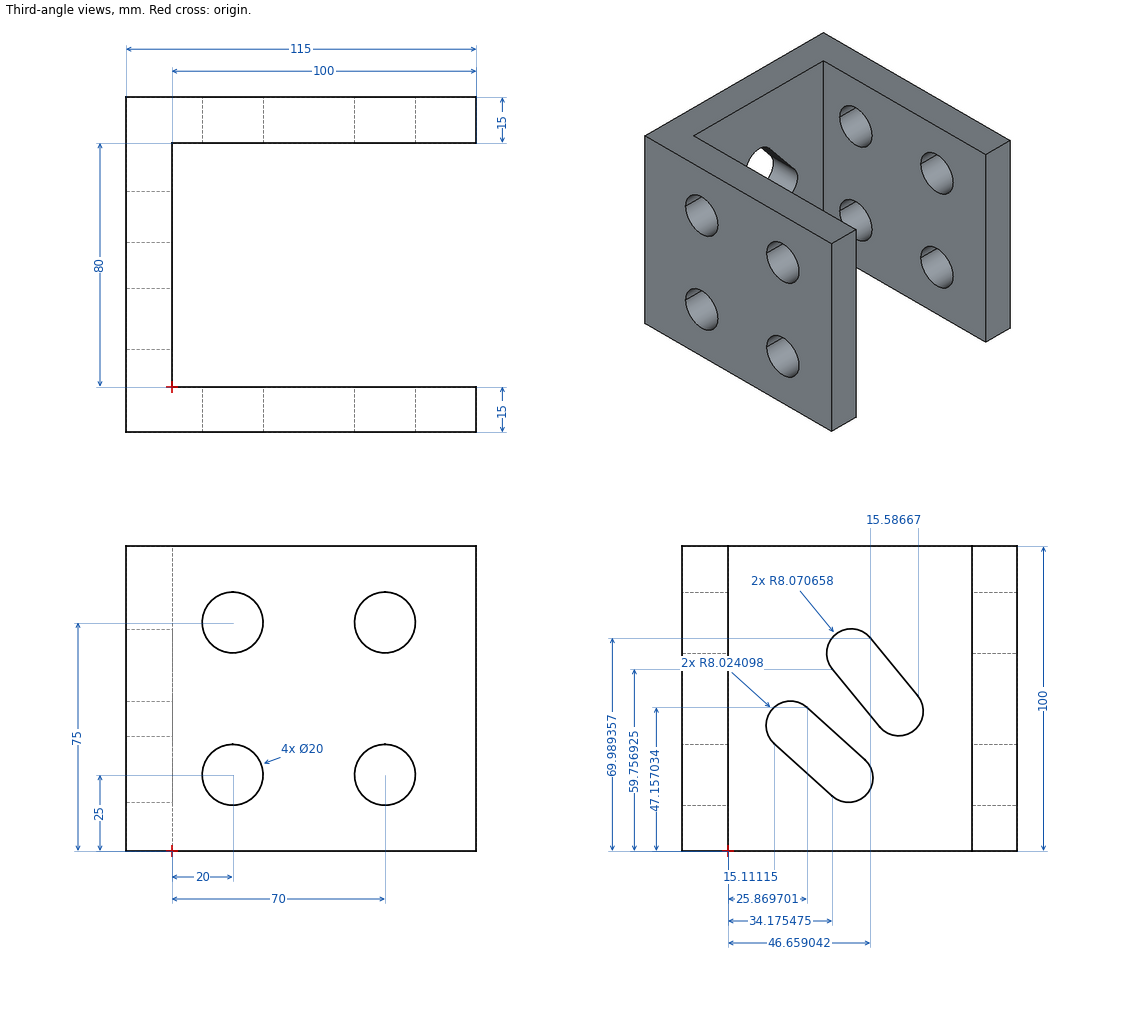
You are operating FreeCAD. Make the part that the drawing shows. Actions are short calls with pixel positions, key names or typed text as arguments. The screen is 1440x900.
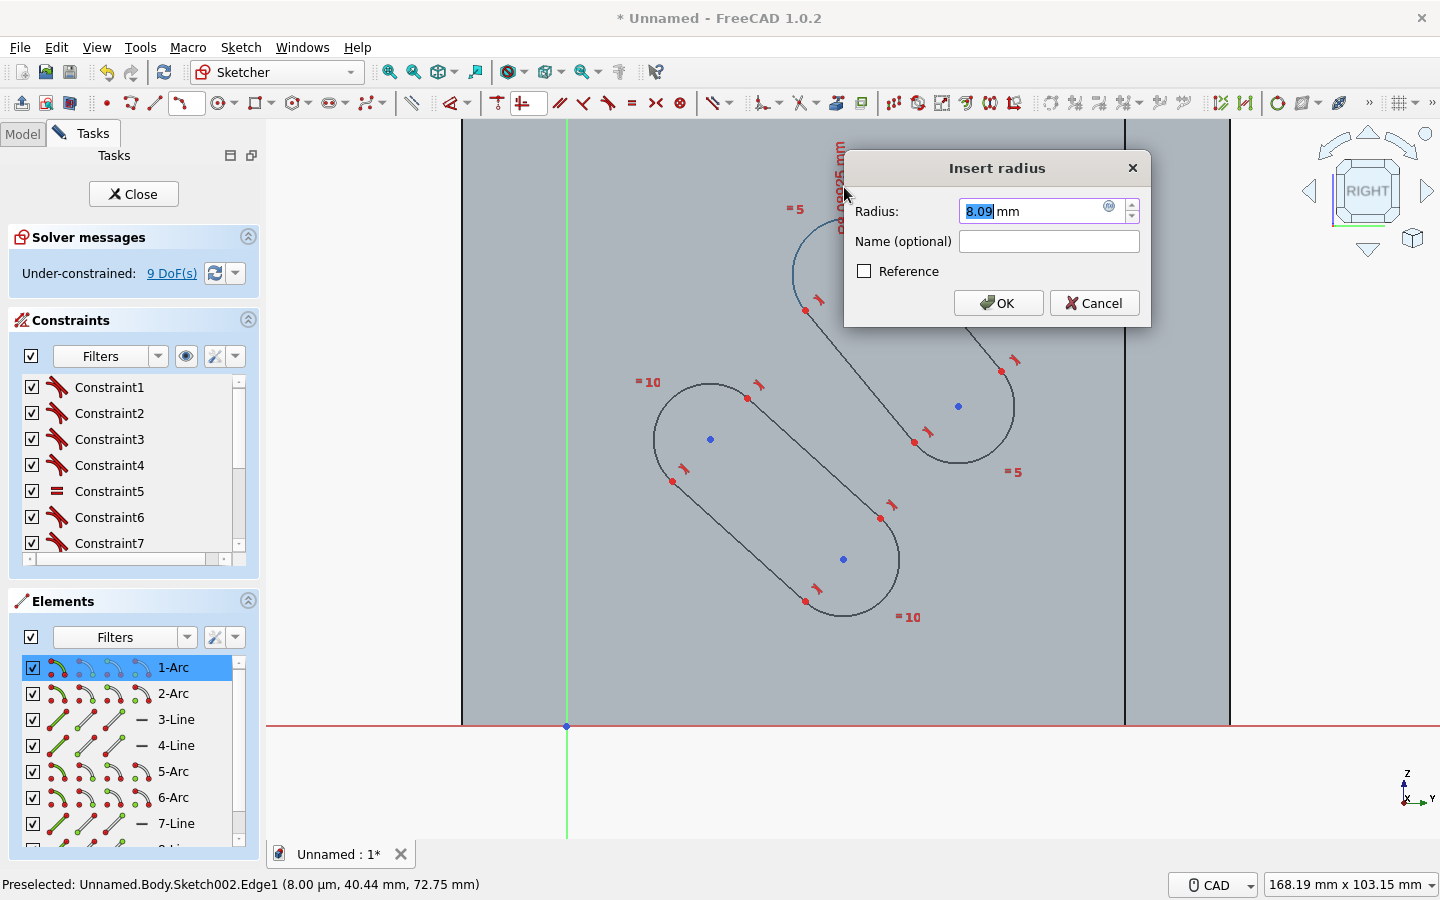
text(8.070658)
key(Return)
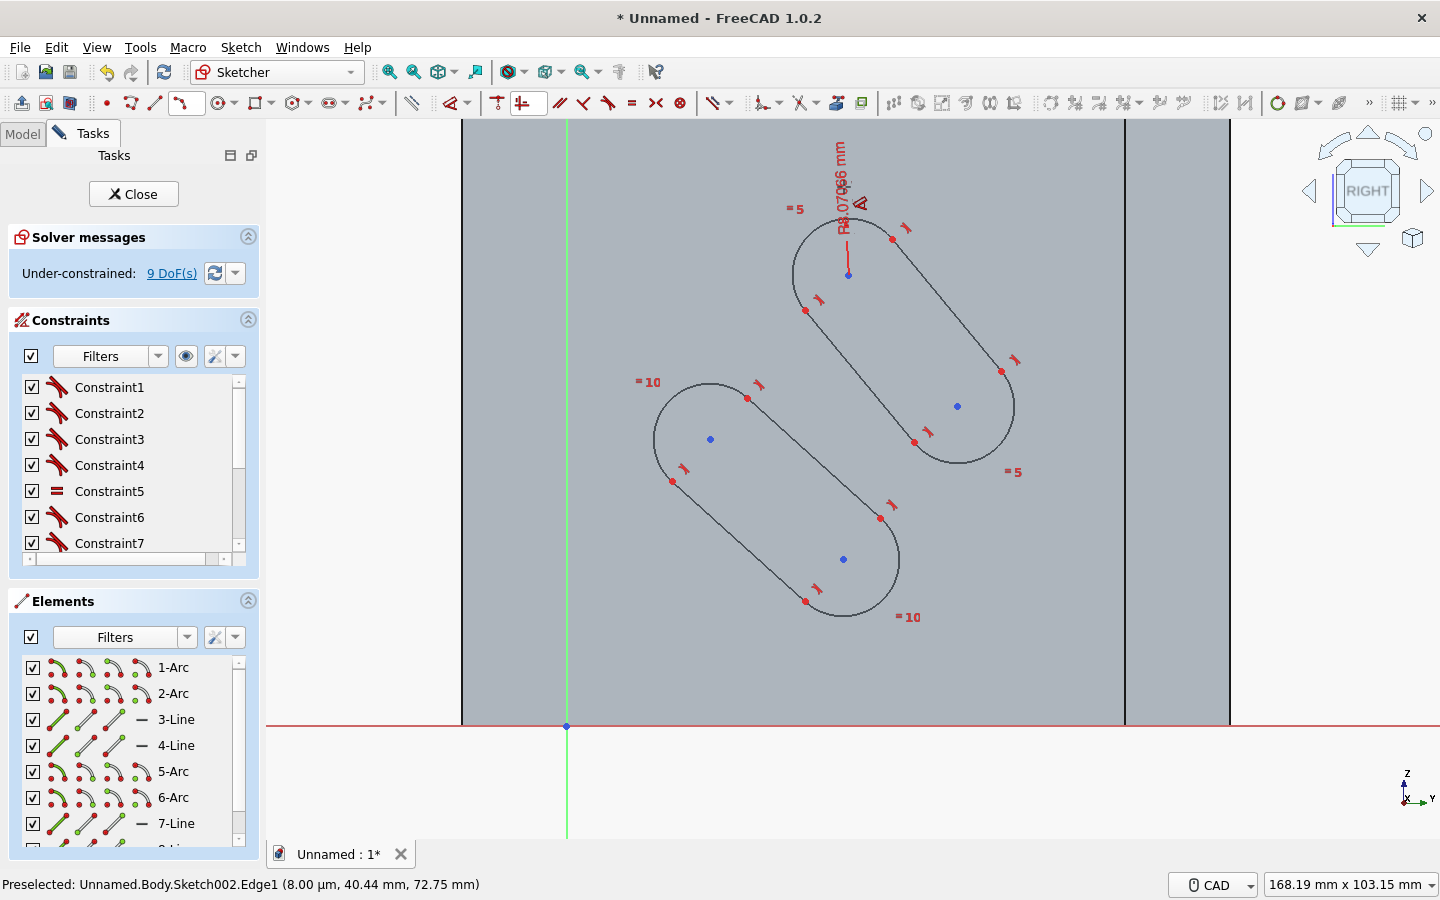
click(698, 385)
click(691, 354)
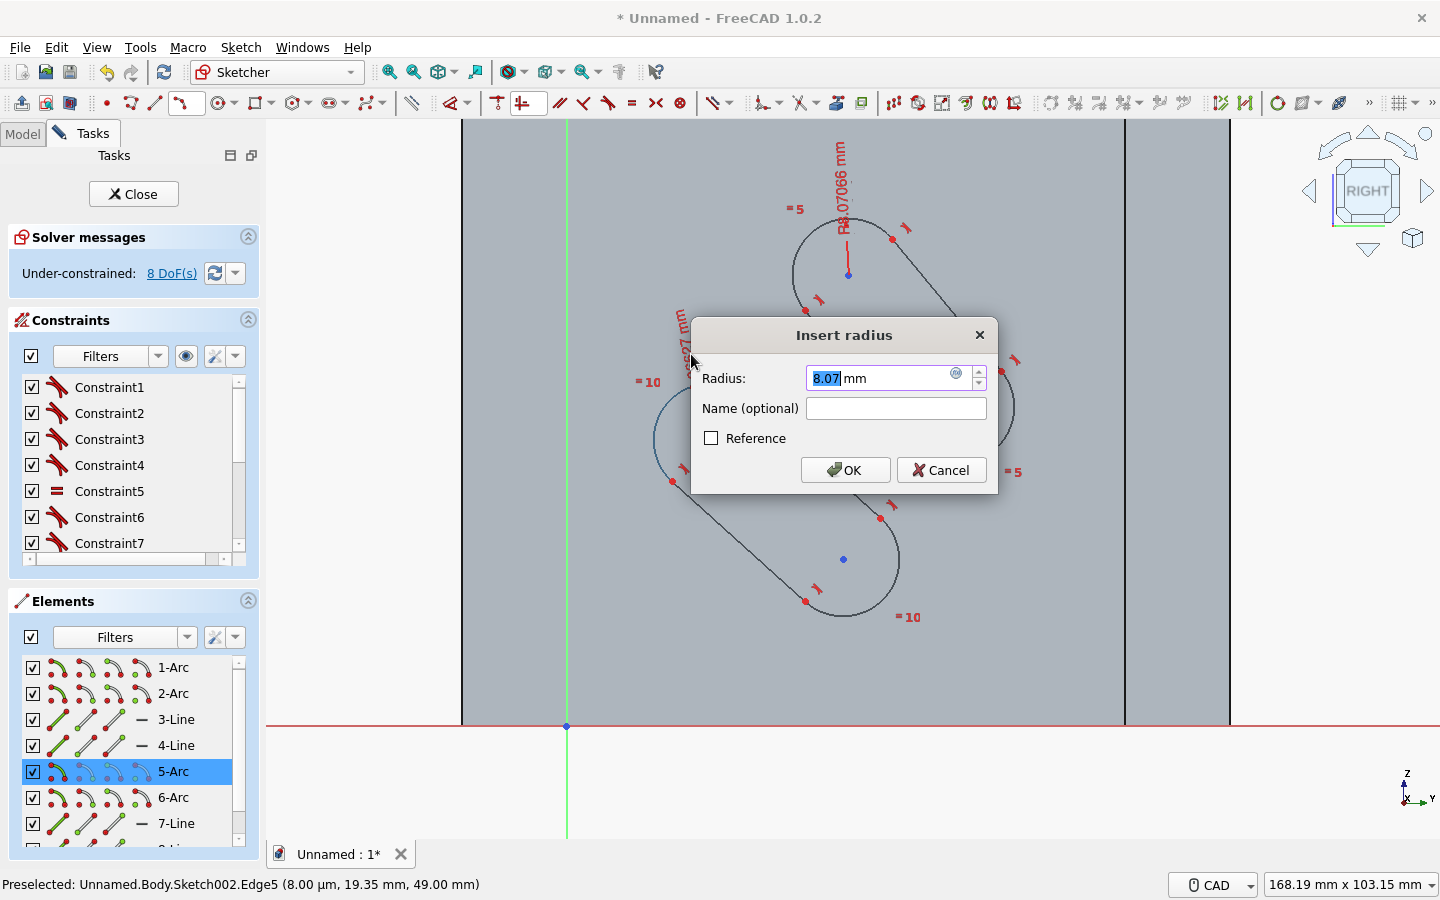
text(8.024098)
key(Return)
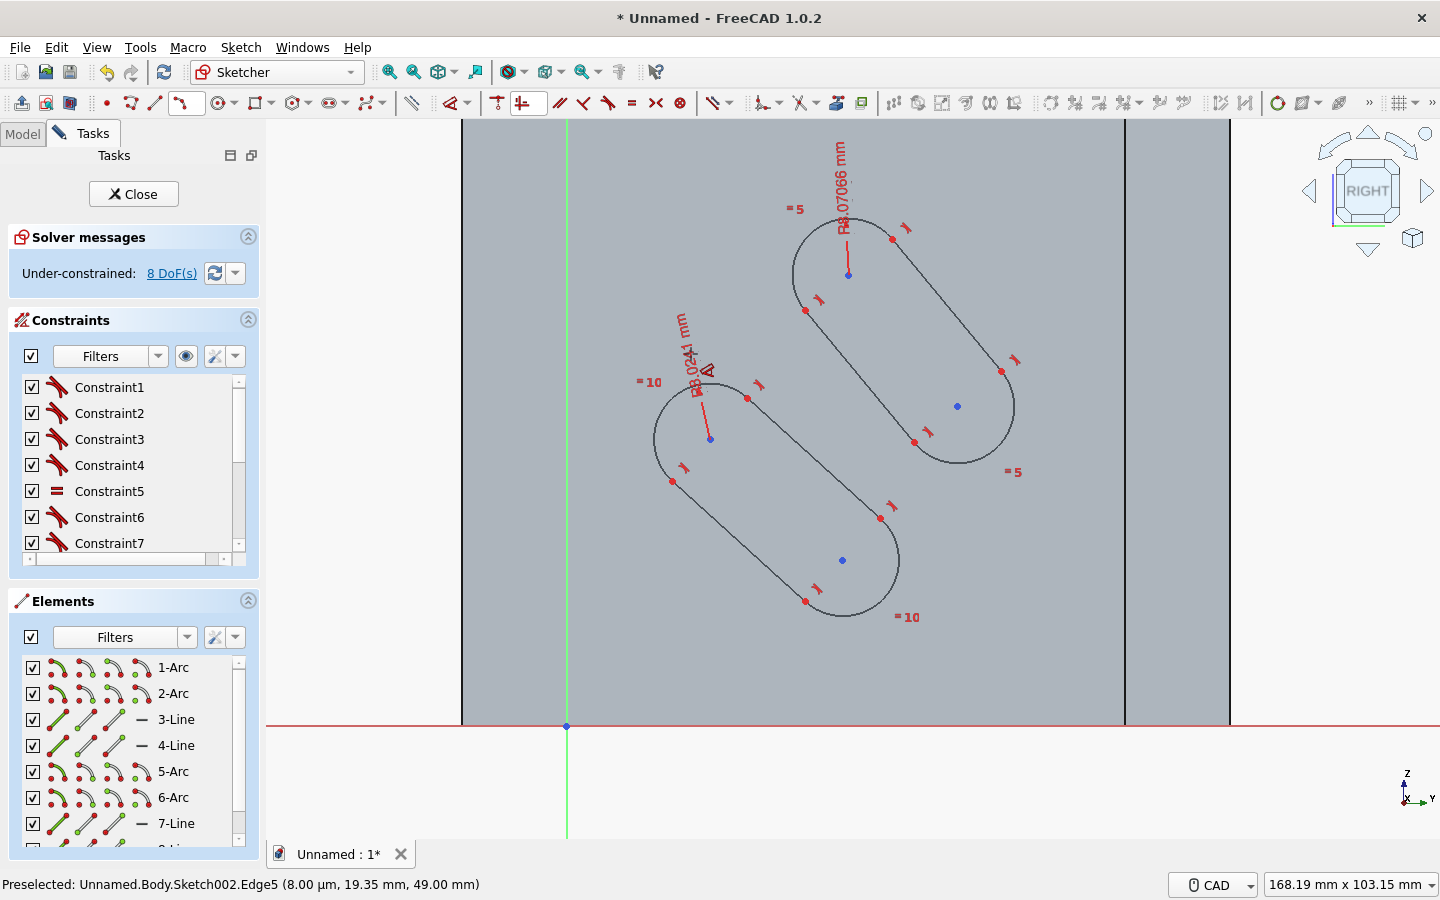
click(672, 481)
click(620, 760)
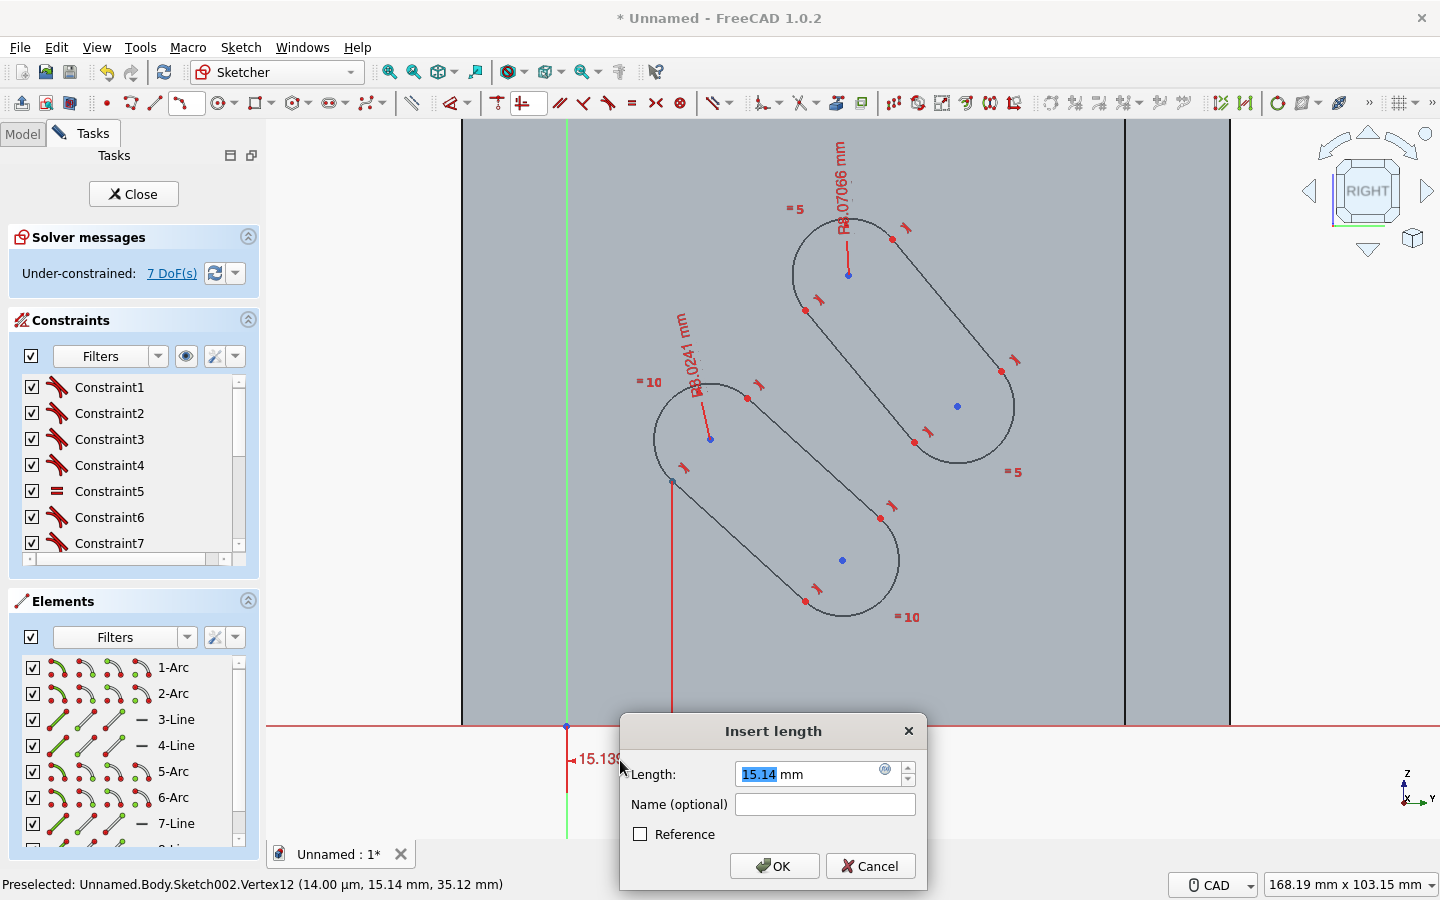
text(15.11115)
key(Return)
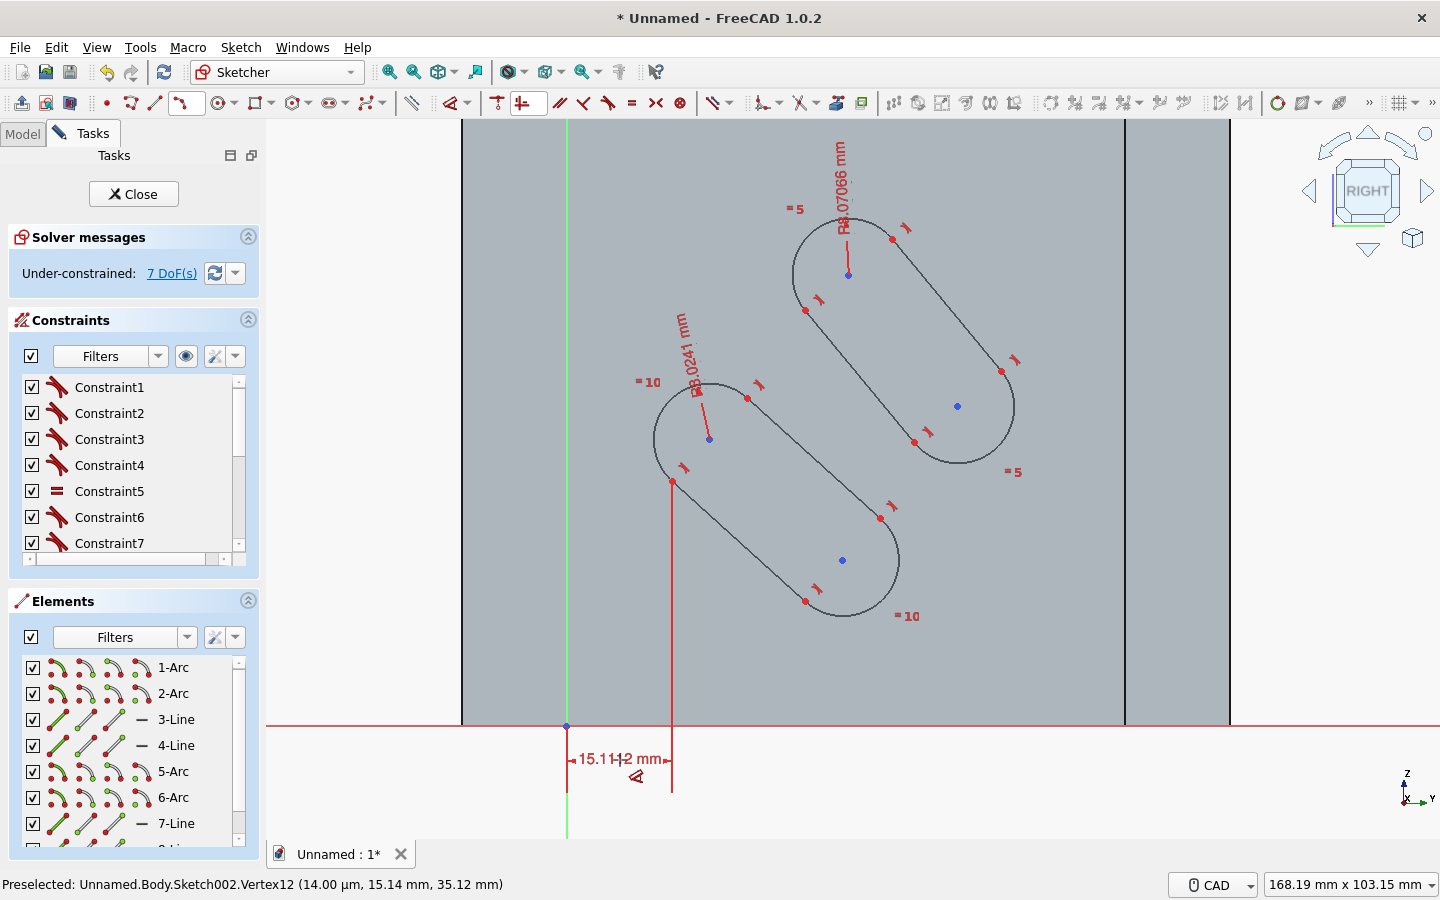
click(925, 279)
click(947, 205)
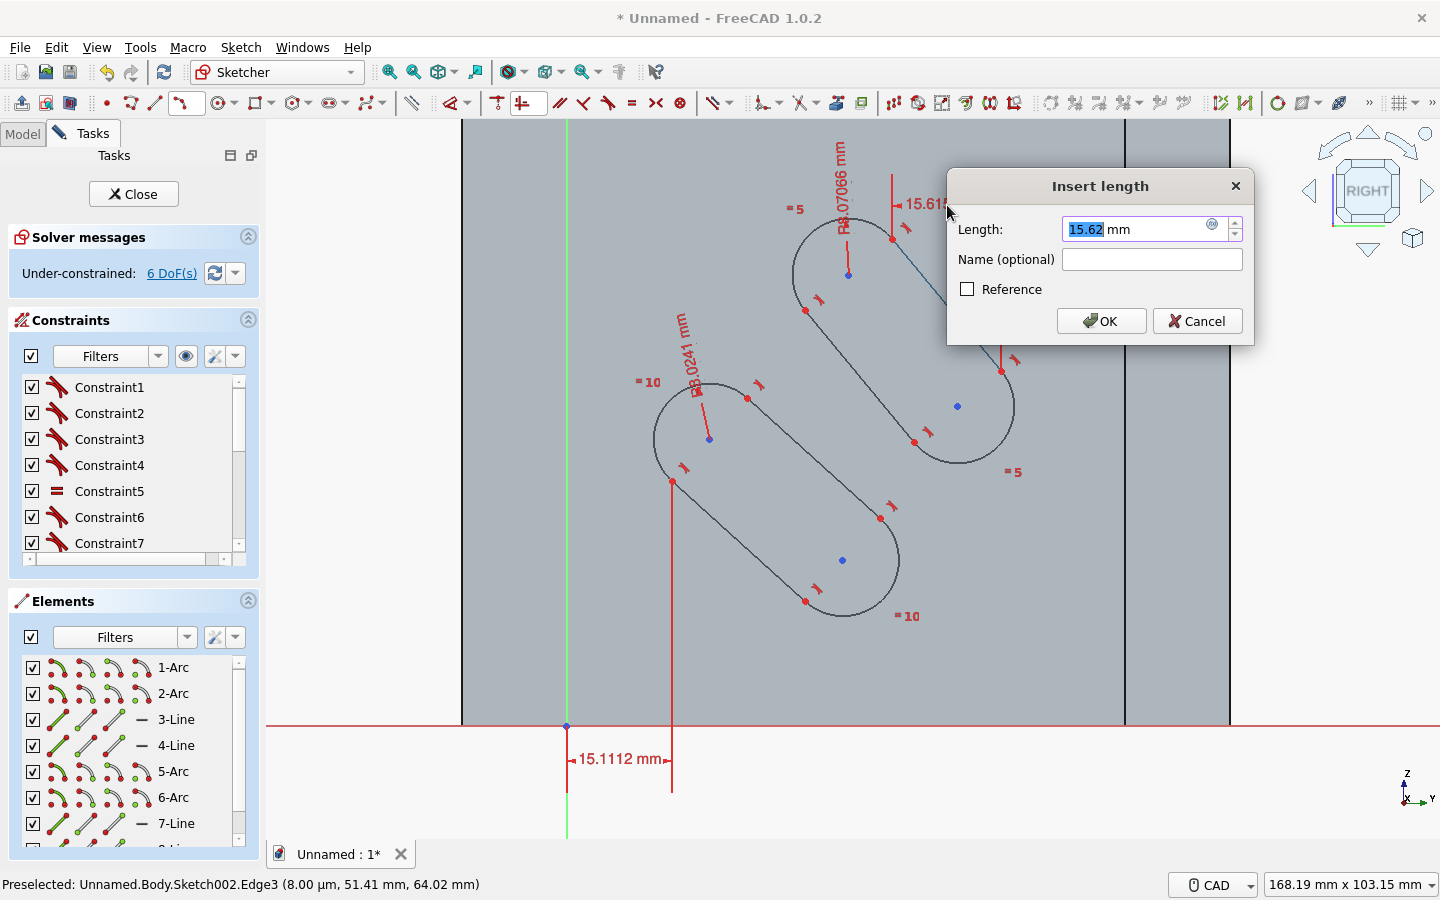
text(15.58667)
key(Return)